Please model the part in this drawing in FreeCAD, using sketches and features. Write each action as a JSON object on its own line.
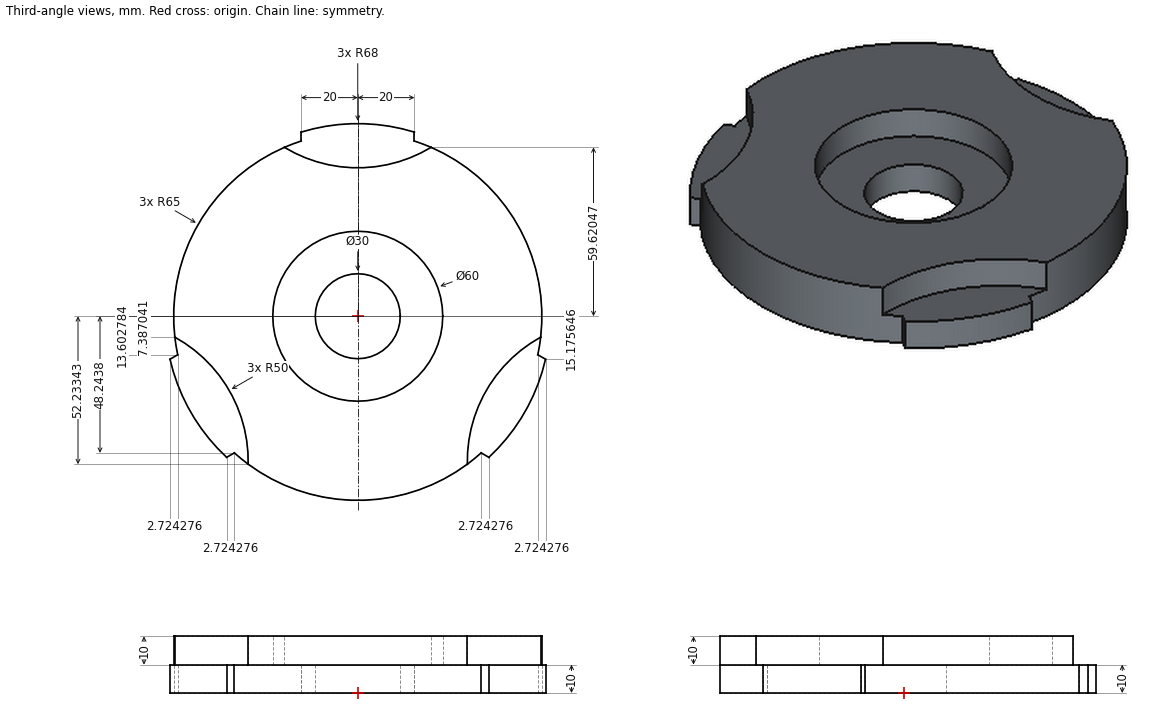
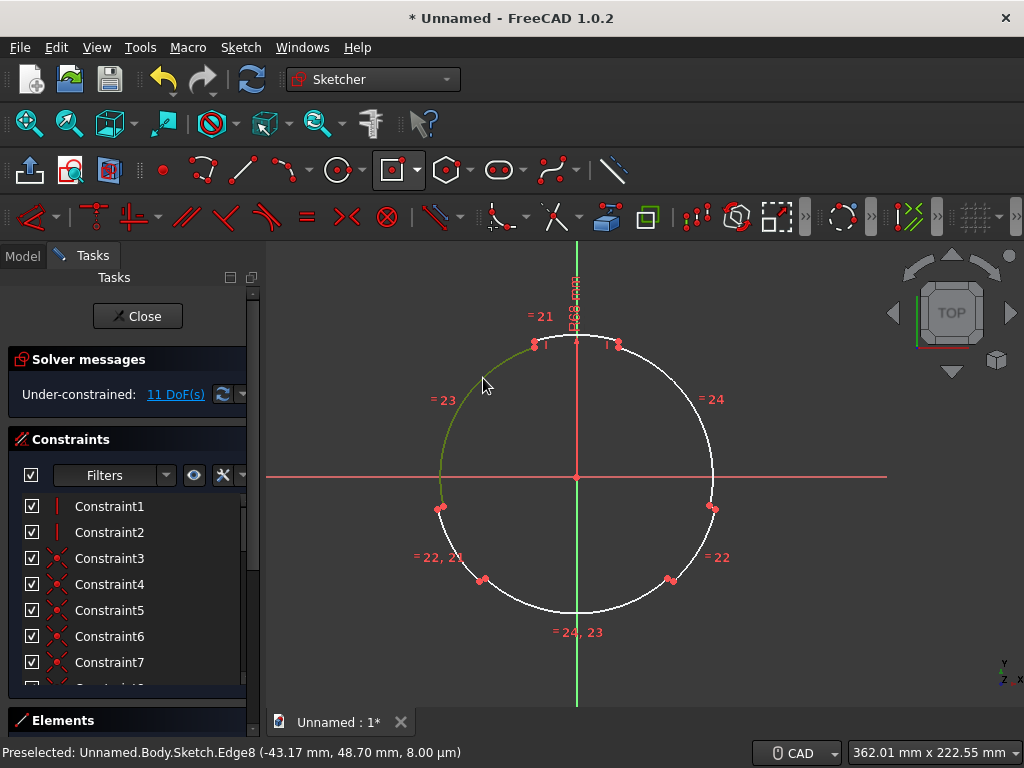
{"action": "key", "text": "k r"}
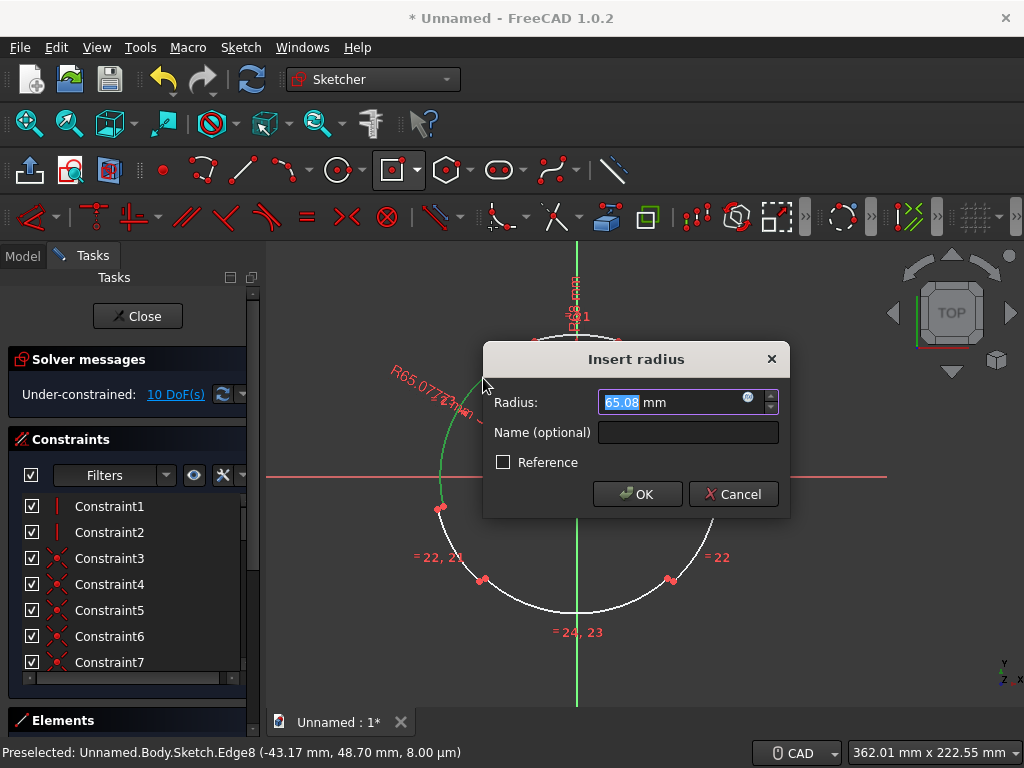
{"action": "type", "text": "65"}
{"action": "key", "text": "Return"}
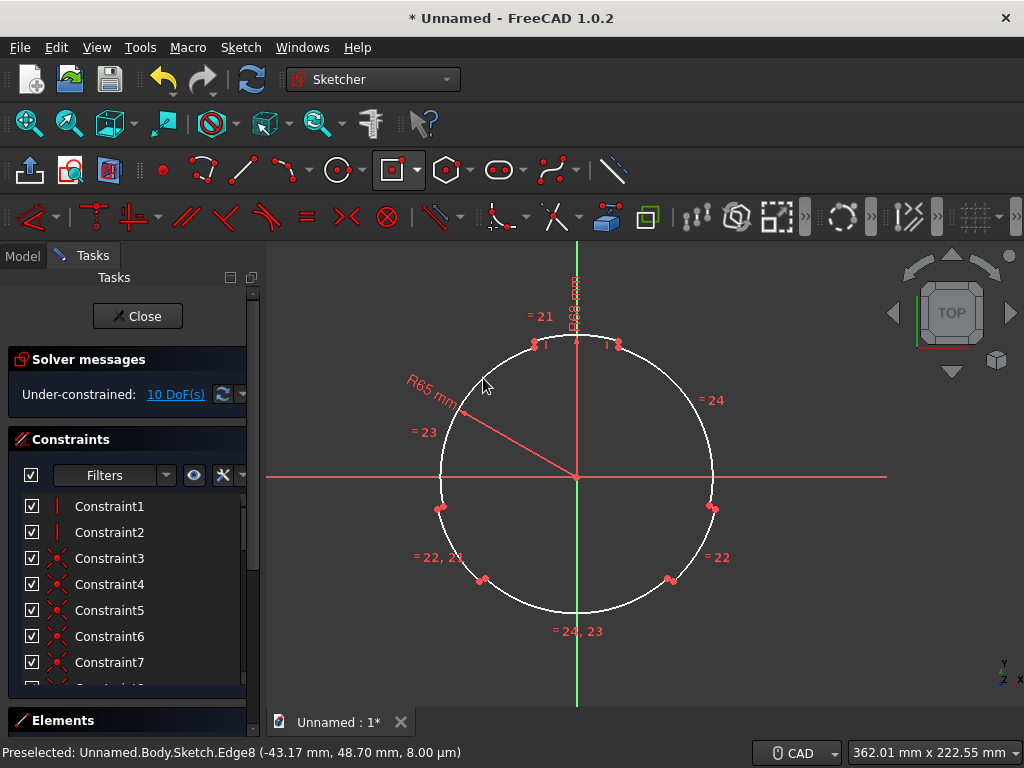
{"action": "scroll", "coordinate": [619, 348], "scroll_direction": "up", "scroll_amount": 4}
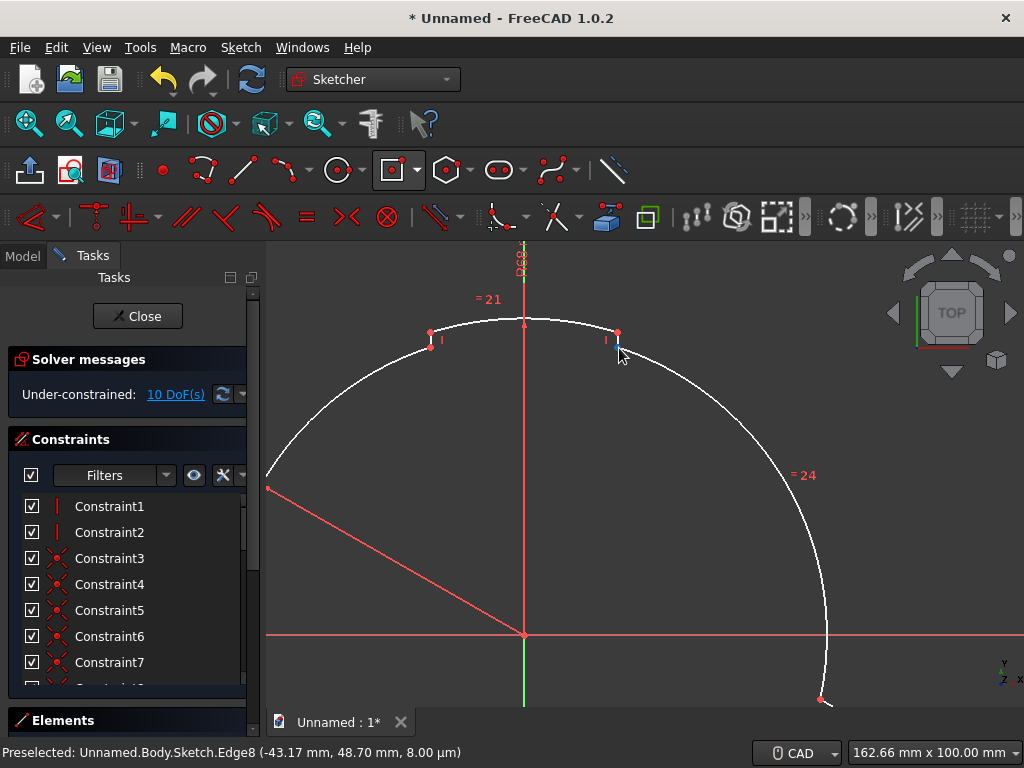
{"action": "left_click", "coordinate": [618, 347]}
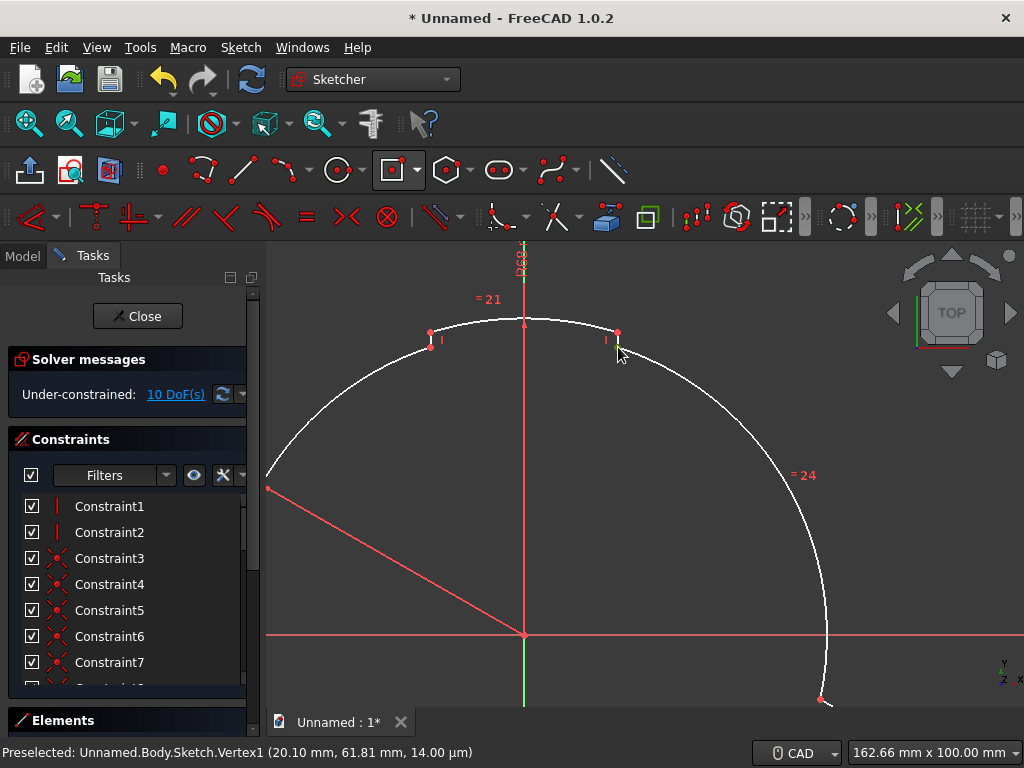
{"action": "key", "text": "l"}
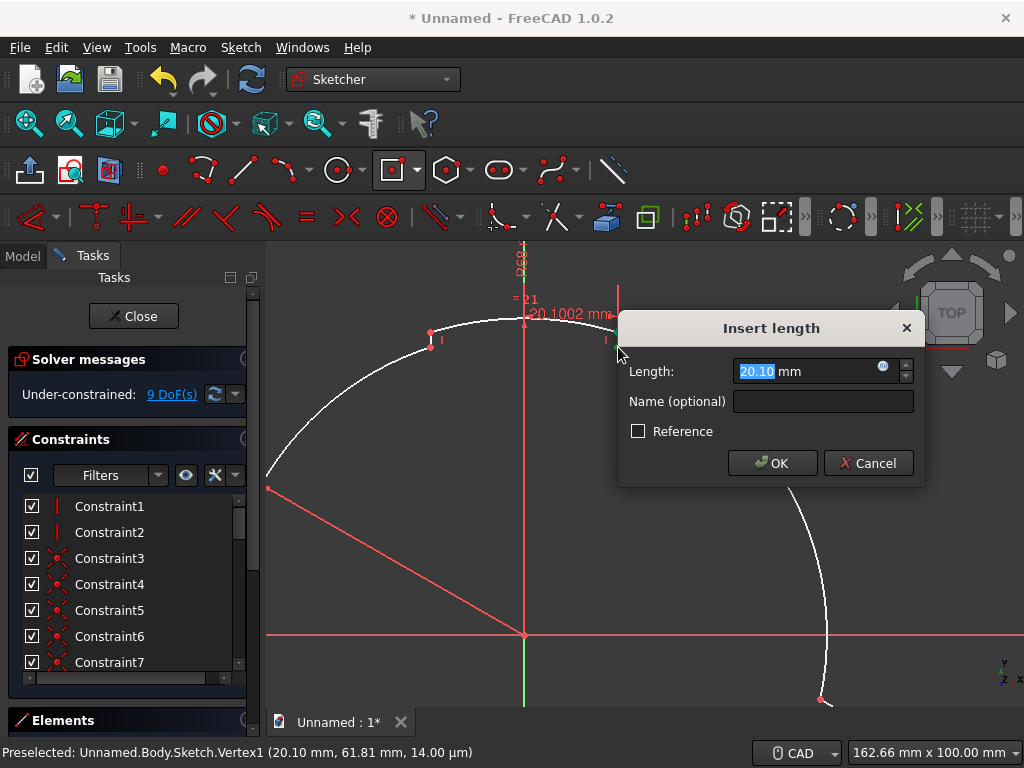
{"action": "type", "text": "20"}
{"action": "key", "text": "Return"}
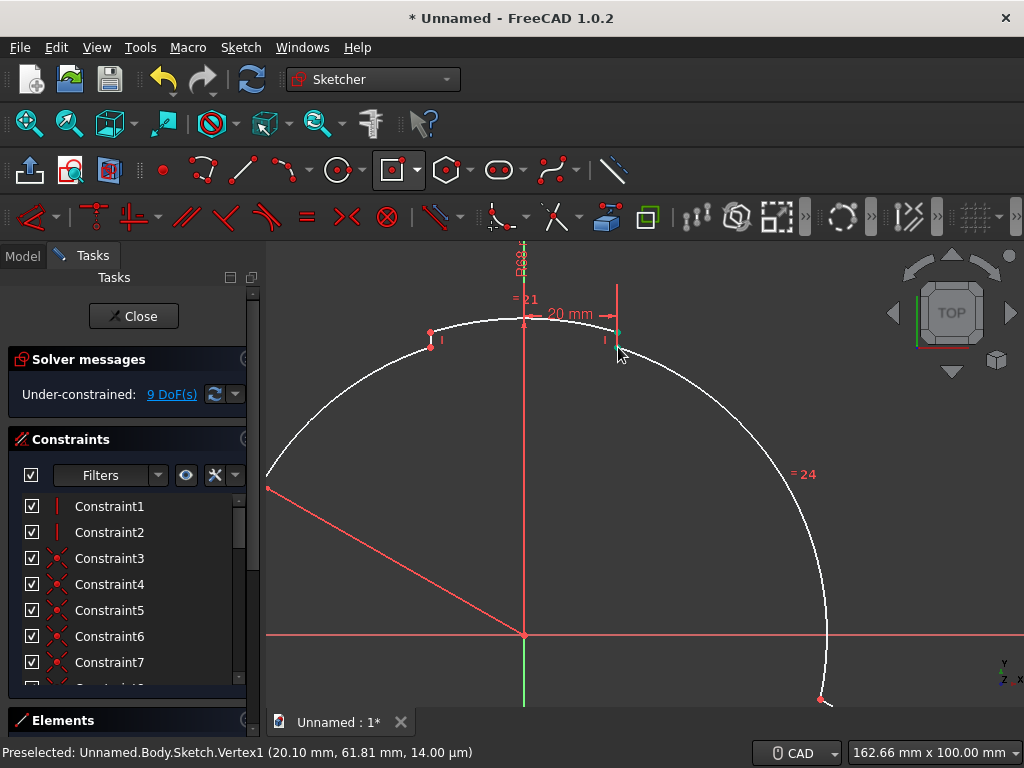
{"action": "left_click", "coordinate": [431, 332]}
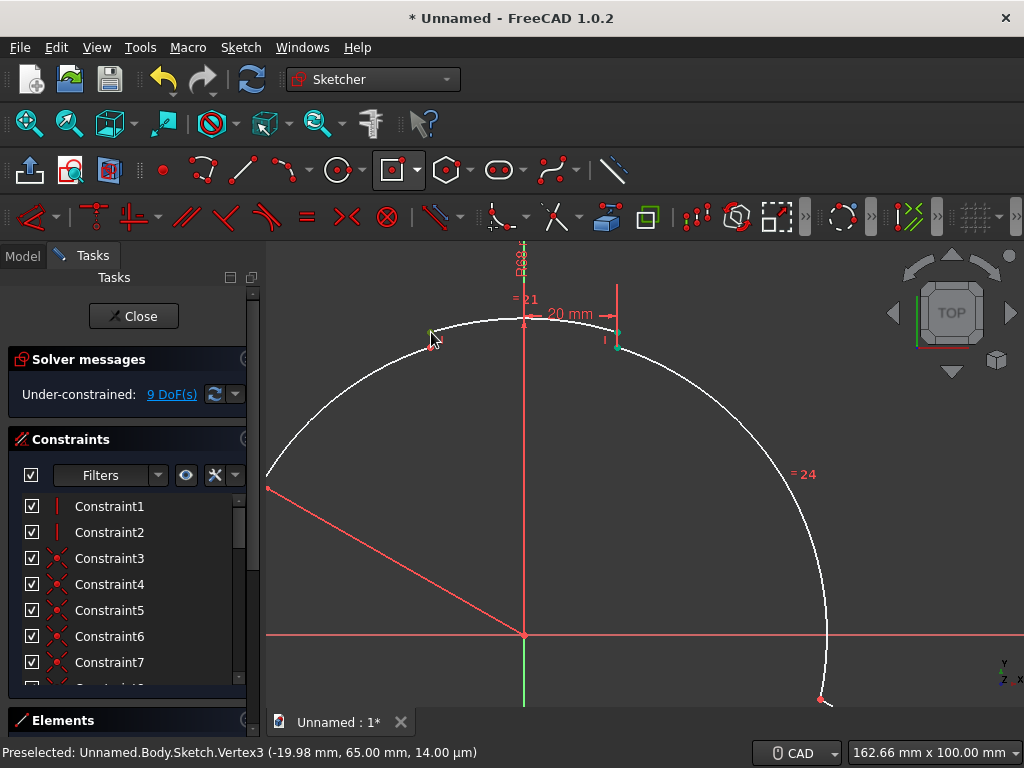
{"action": "key", "text": "l"}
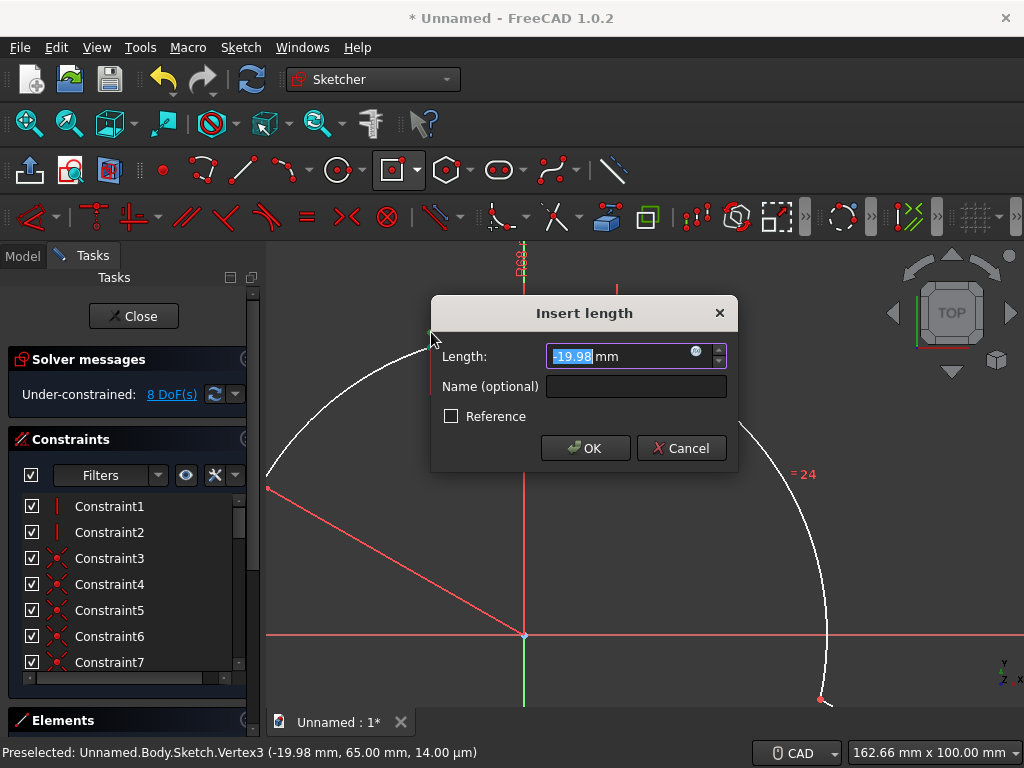
{"action": "type", "text": "-20"}
{"action": "key", "text": "Return"}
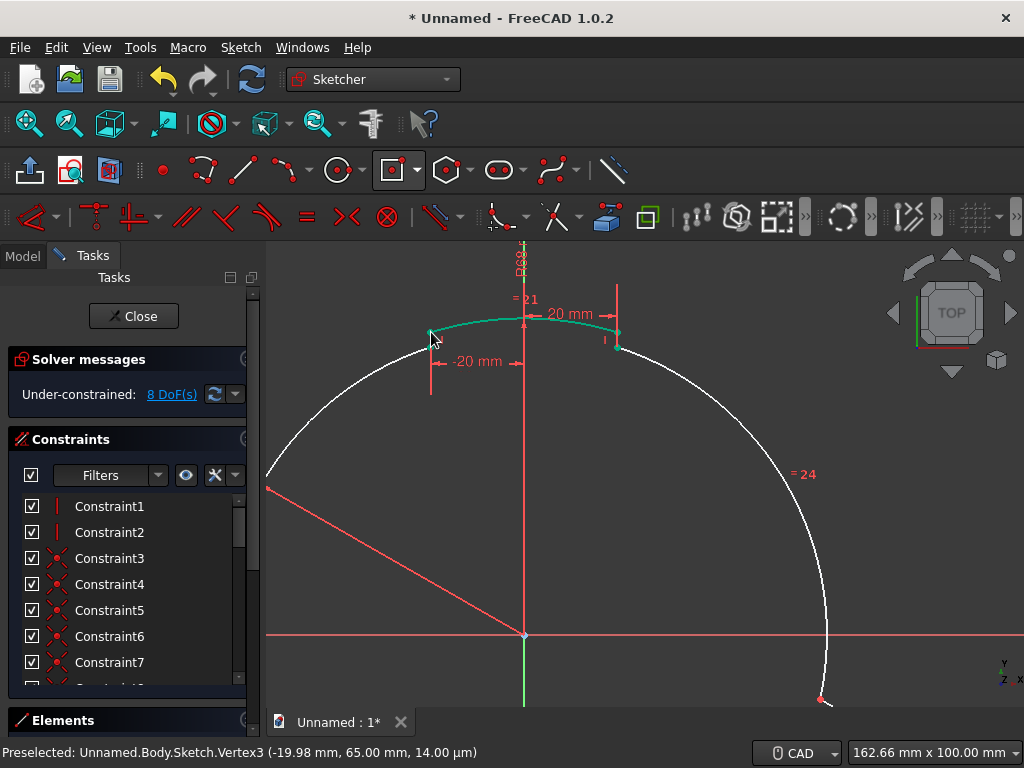
{"action": "scroll", "coordinate": [619, 348], "scroll_direction": "down", "scroll_amount": 4}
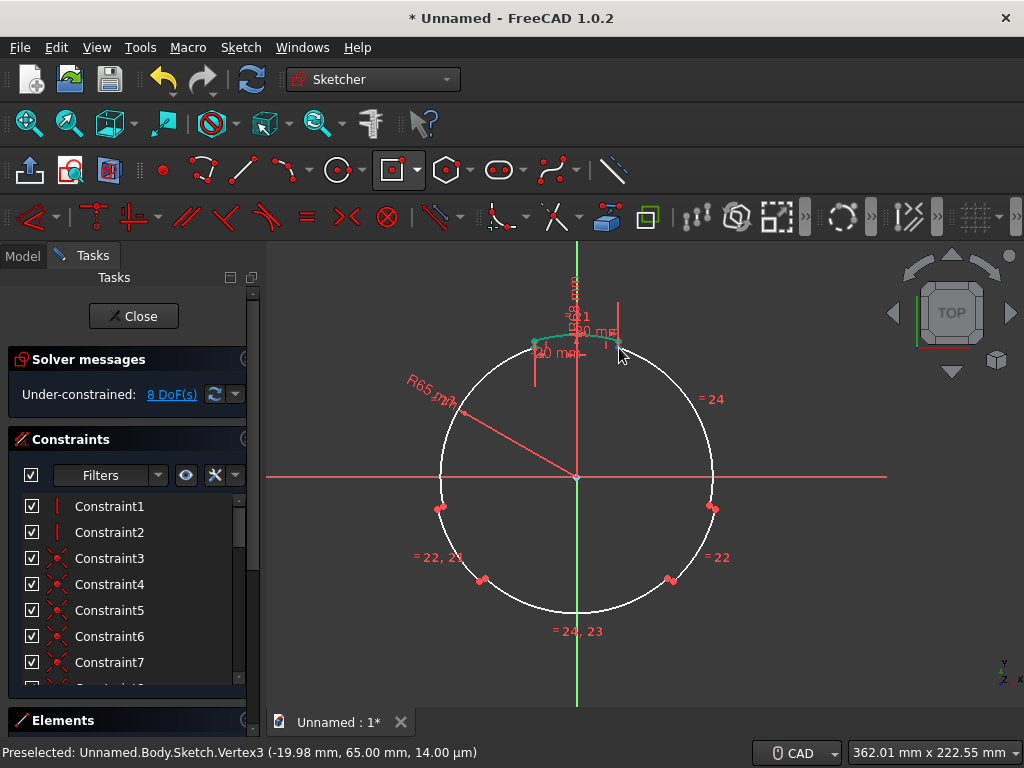
{"action": "scroll", "coordinate": [486, 578], "scroll_direction": "up", "scroll_amount": 4}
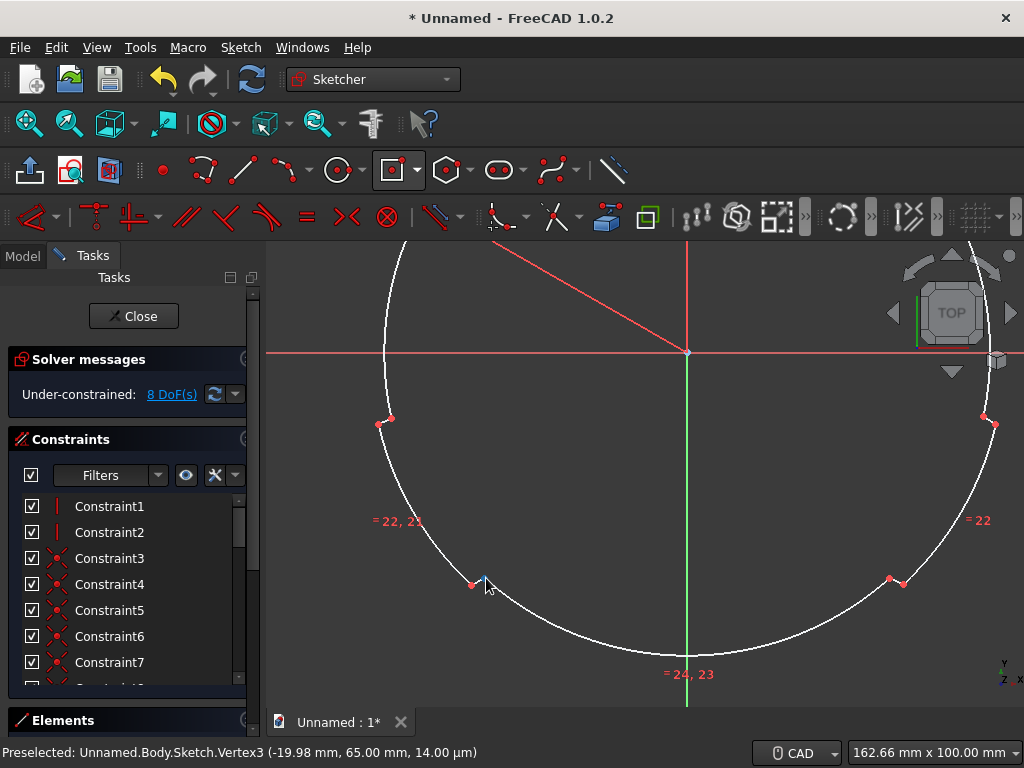
{"action": "left_click", "coordinate": [485, 578]}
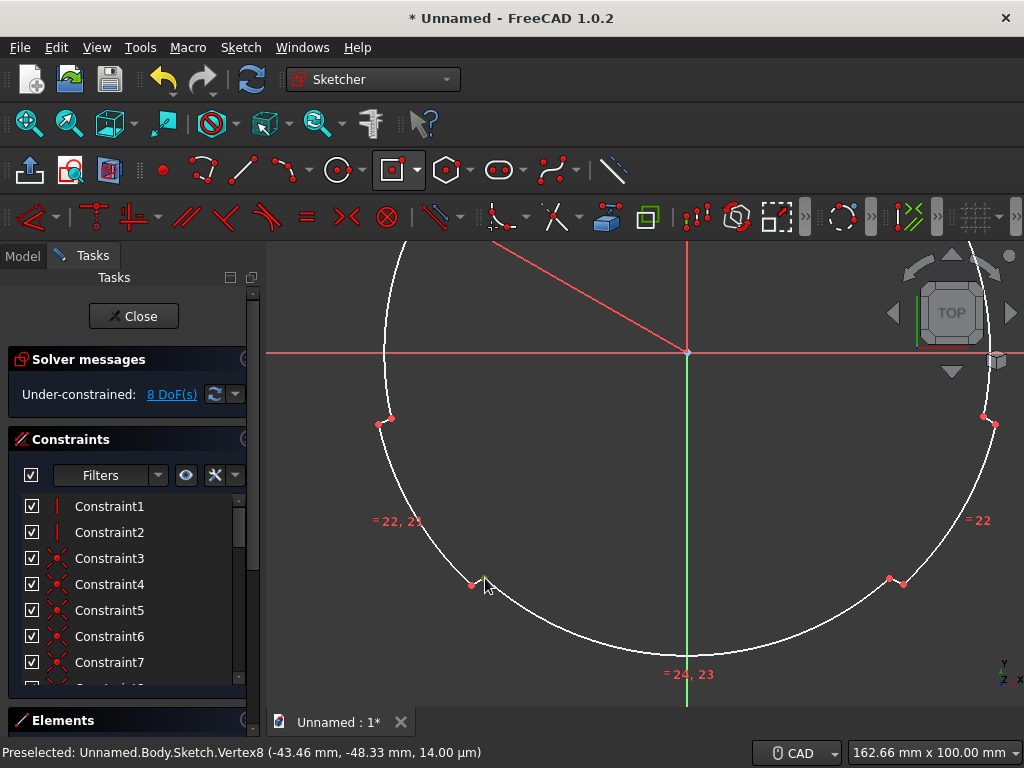
{"action": "key", "text": "i"}